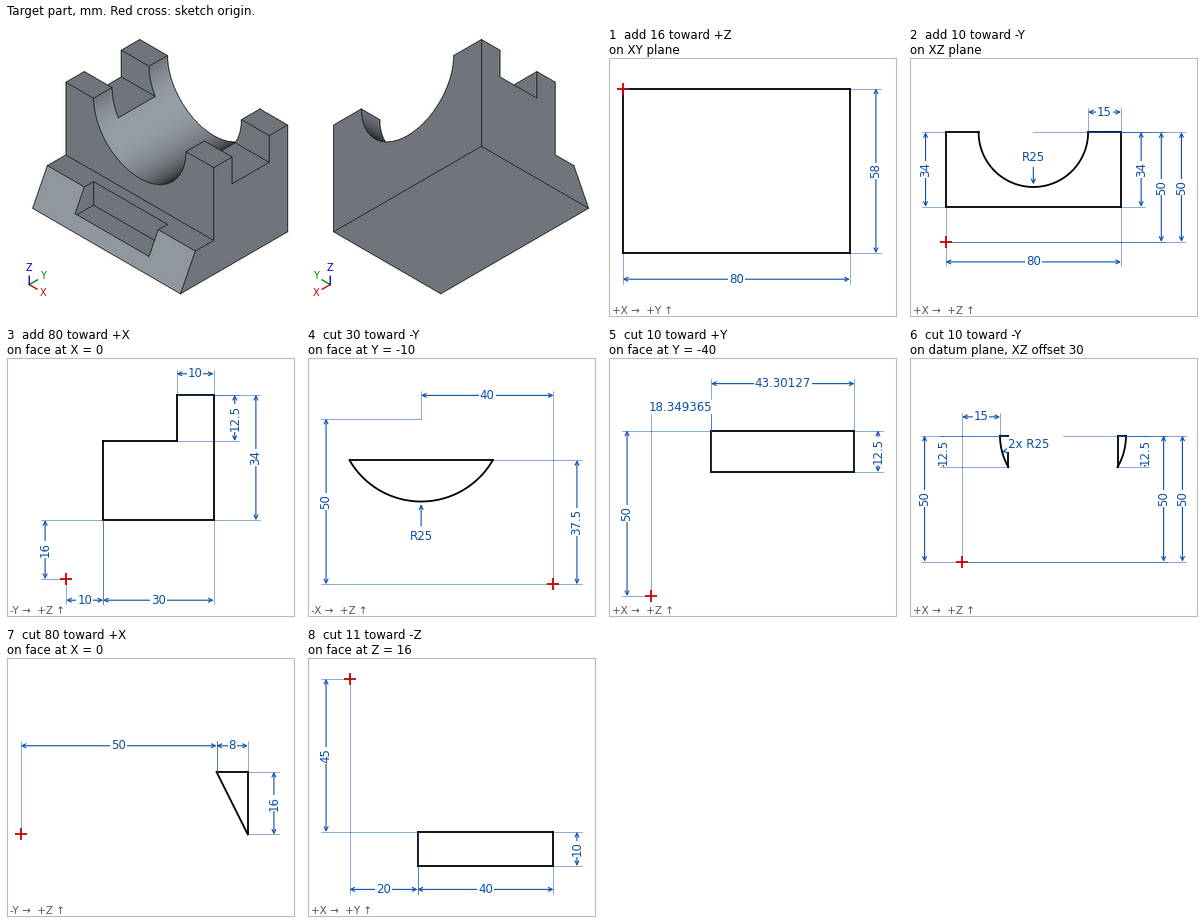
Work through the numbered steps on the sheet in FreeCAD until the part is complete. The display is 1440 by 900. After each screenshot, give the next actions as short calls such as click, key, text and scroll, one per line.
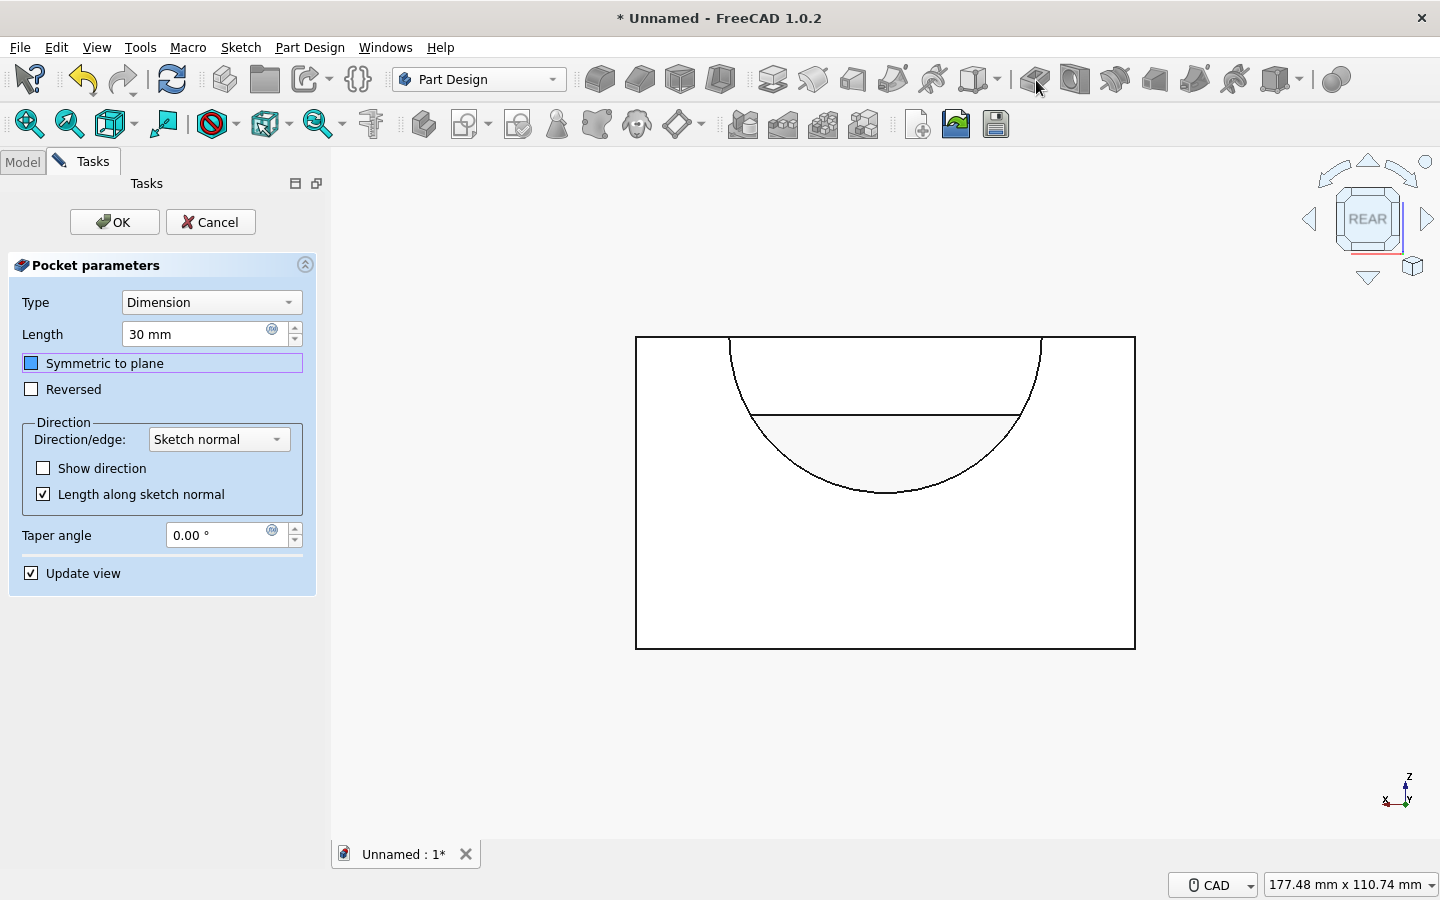
click(115, 222)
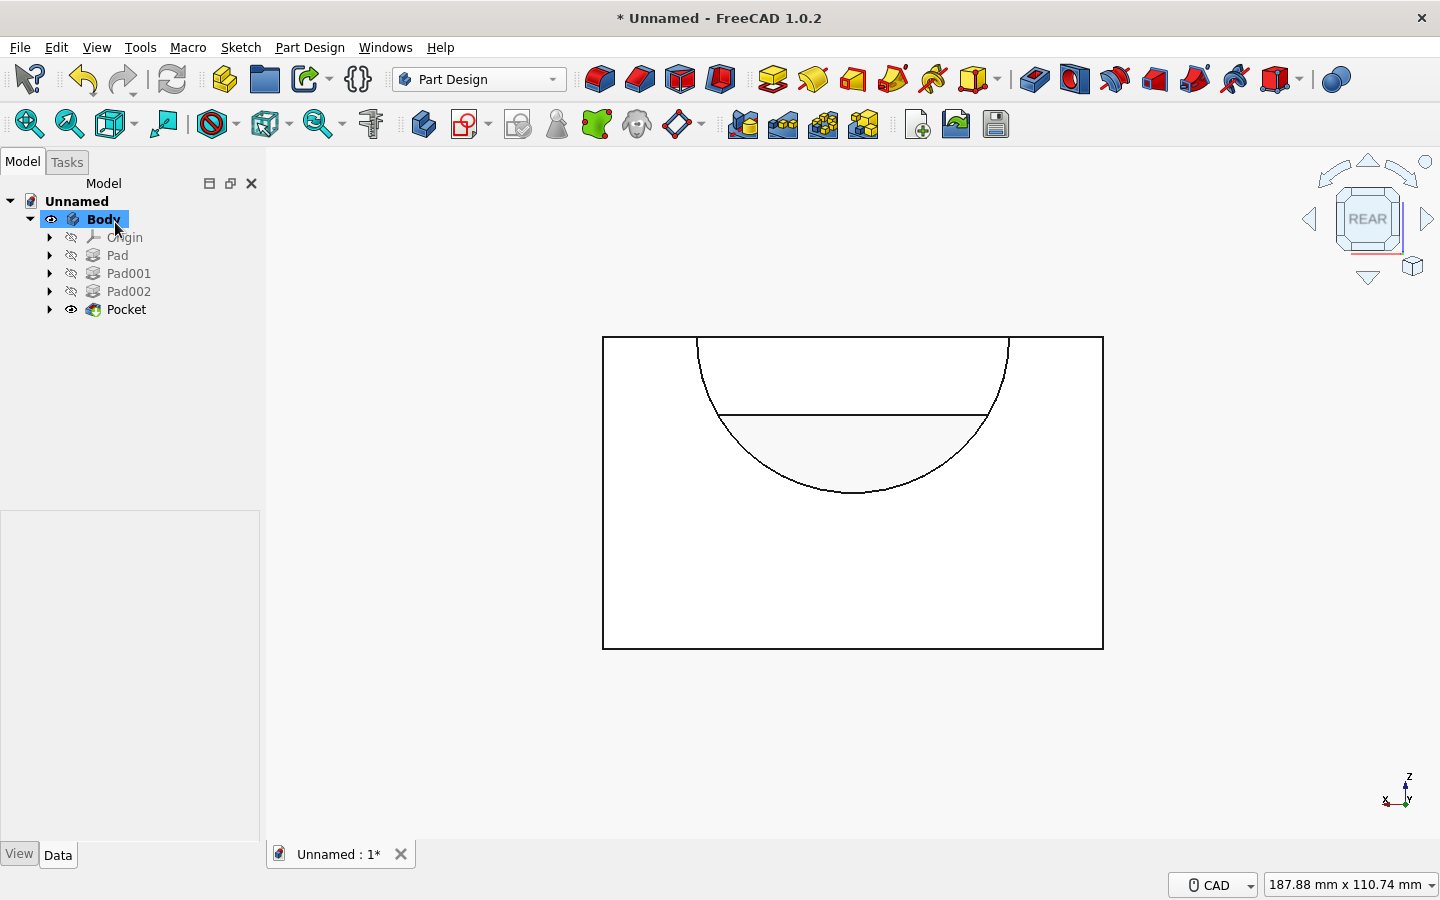
key(0)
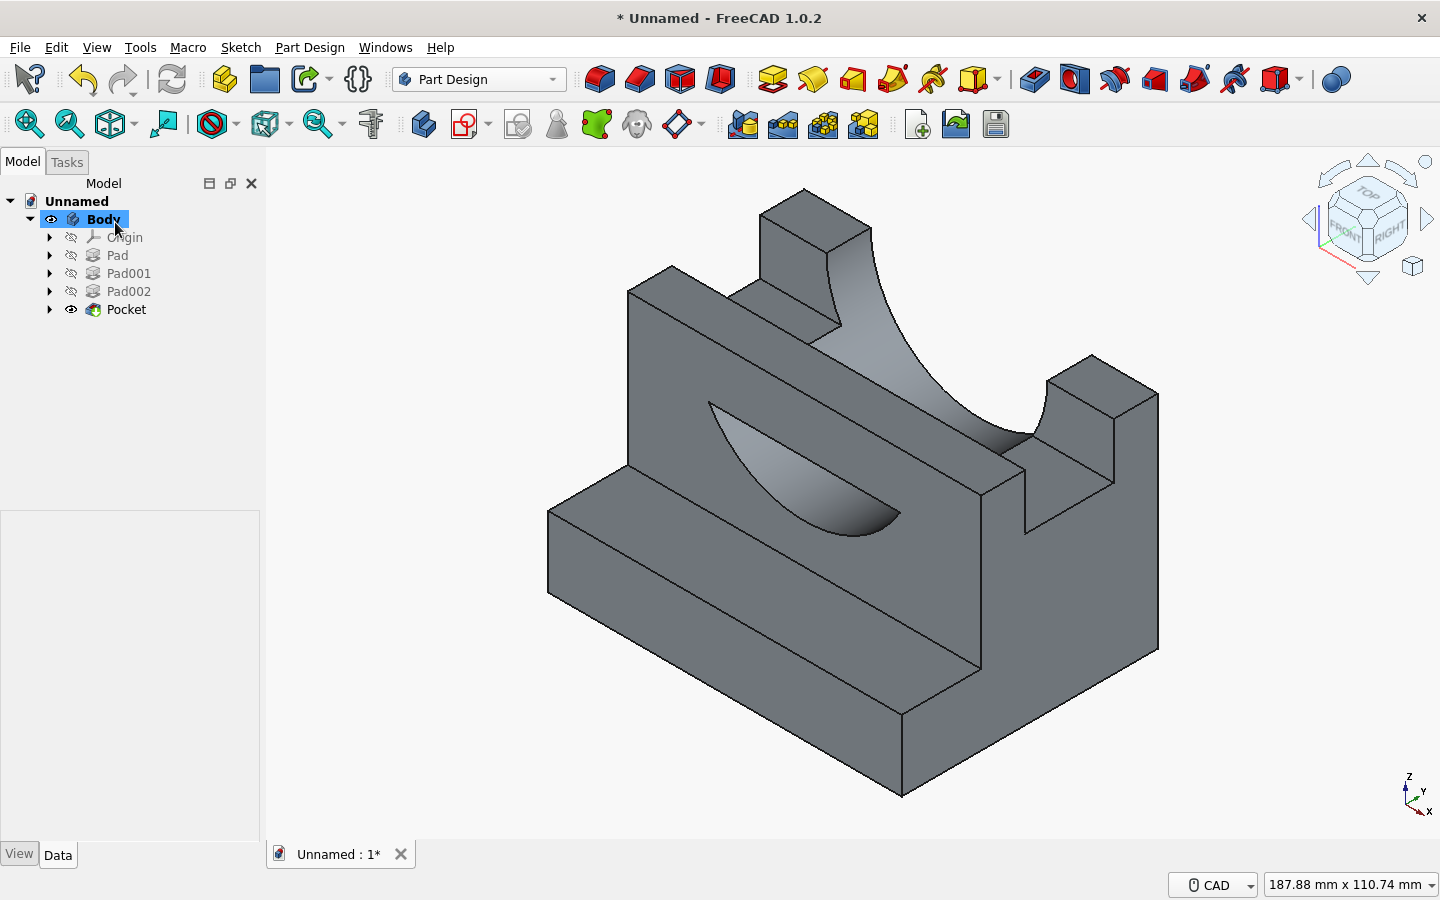
click(905, 587)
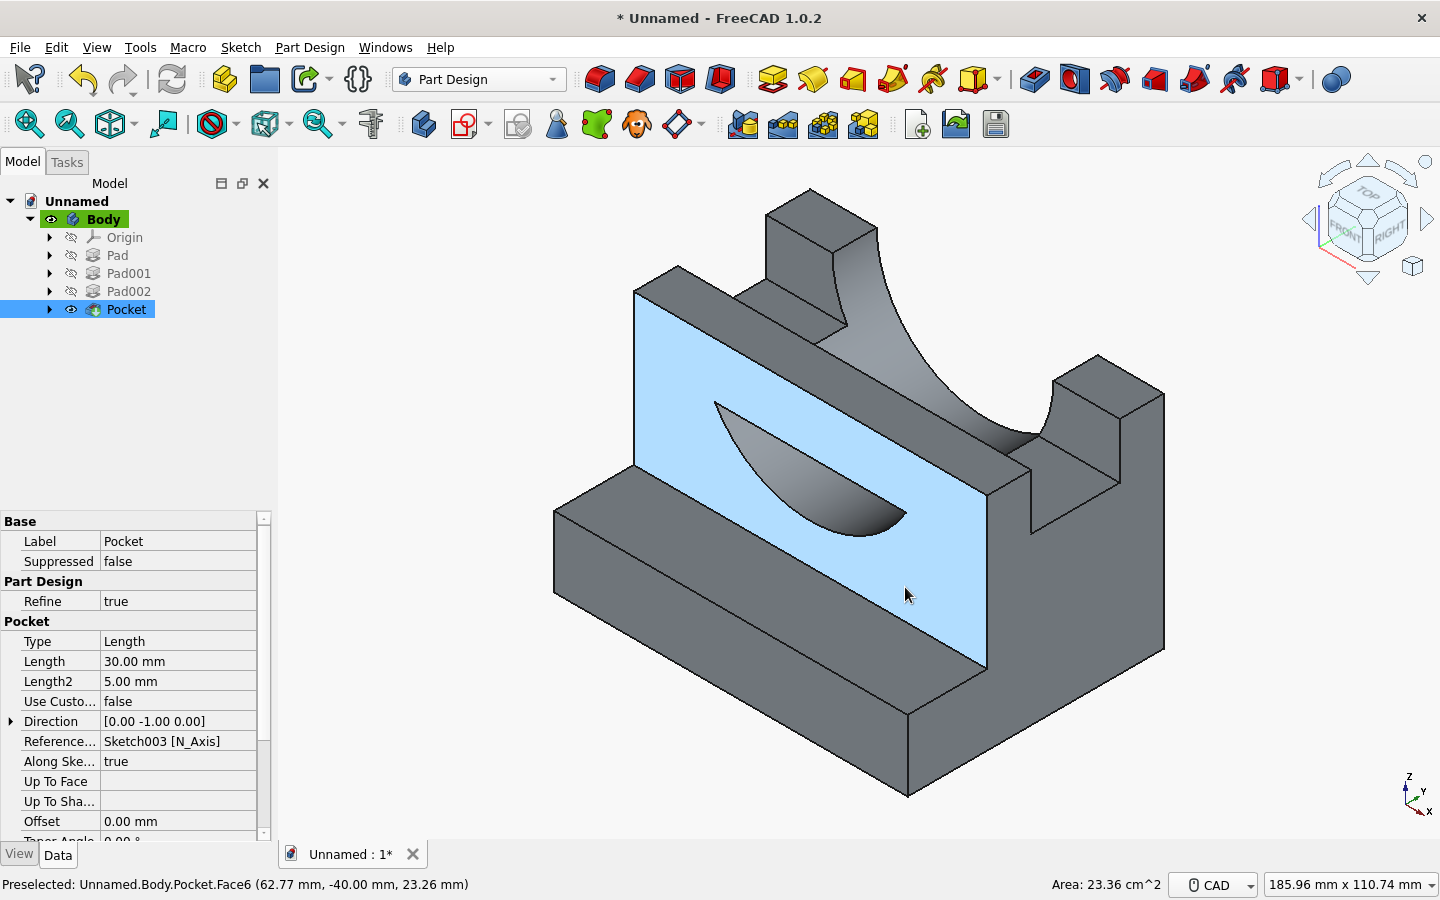
click(464, 124)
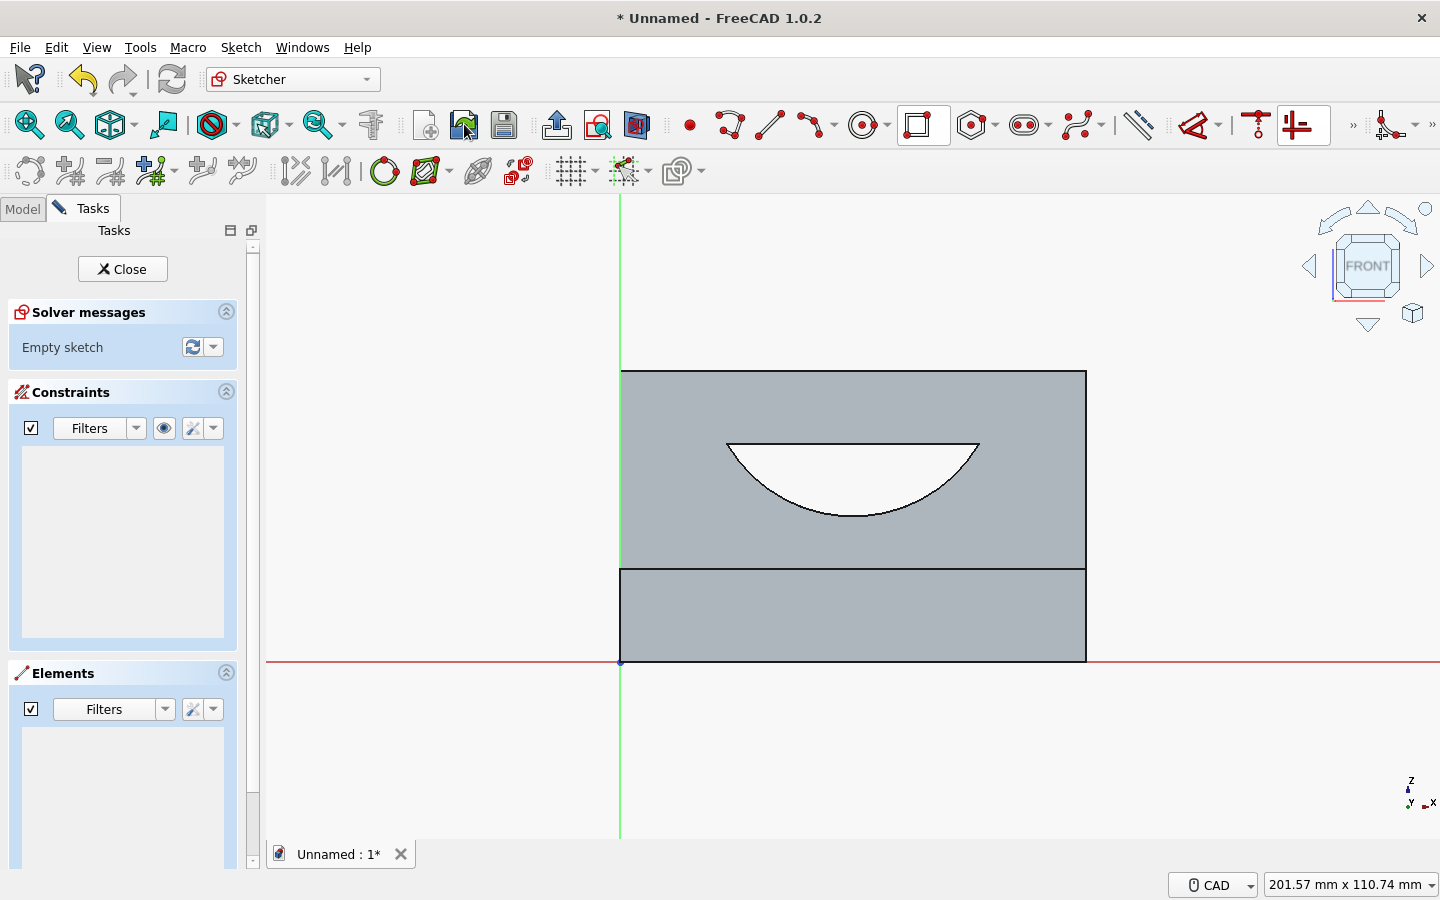
scroll(830, 517, up, 2)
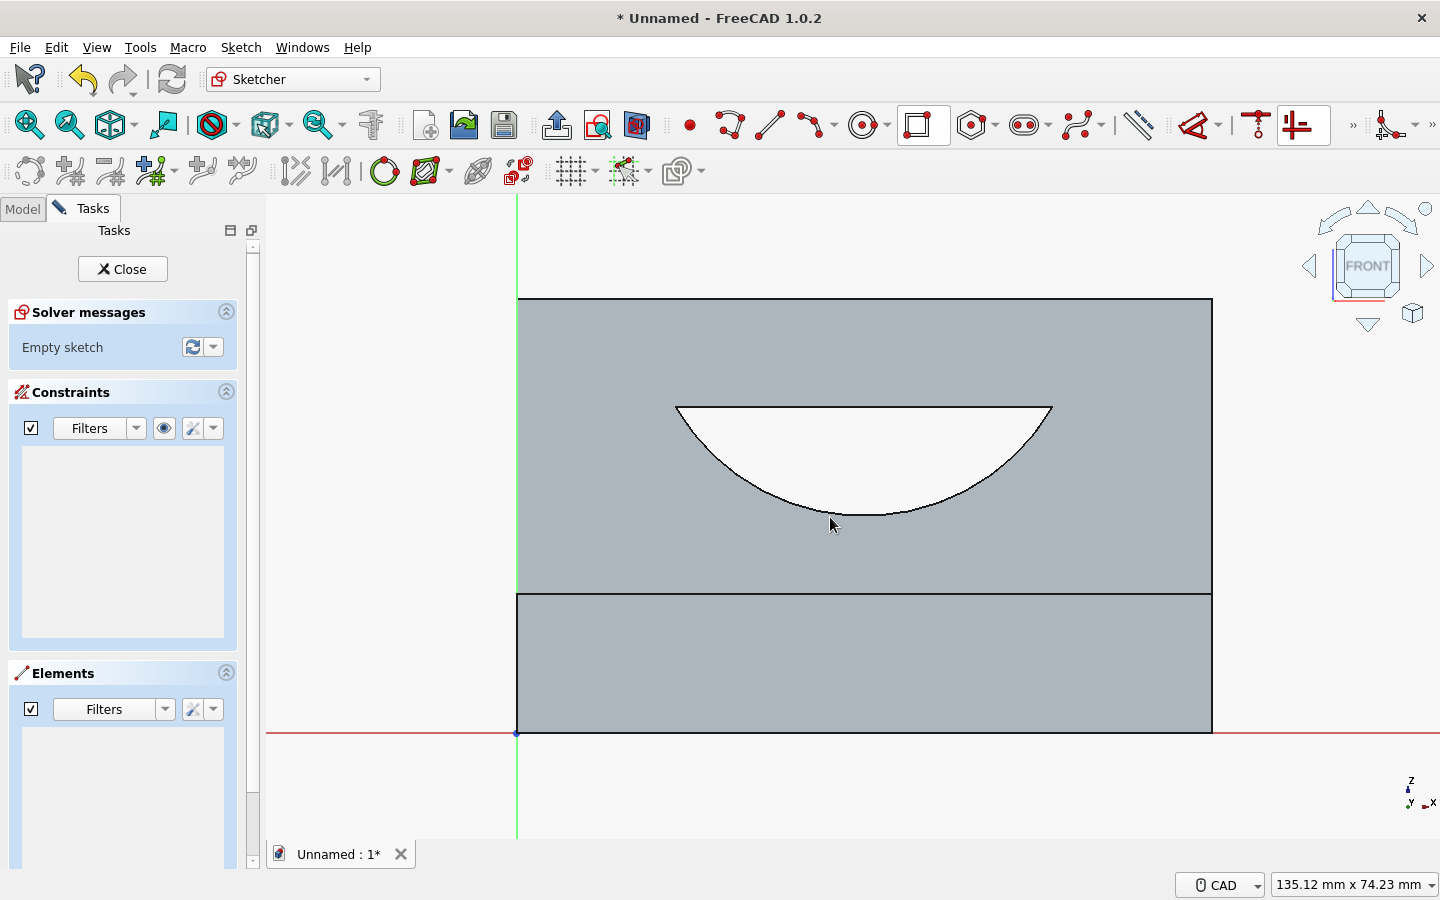
click(918, 126)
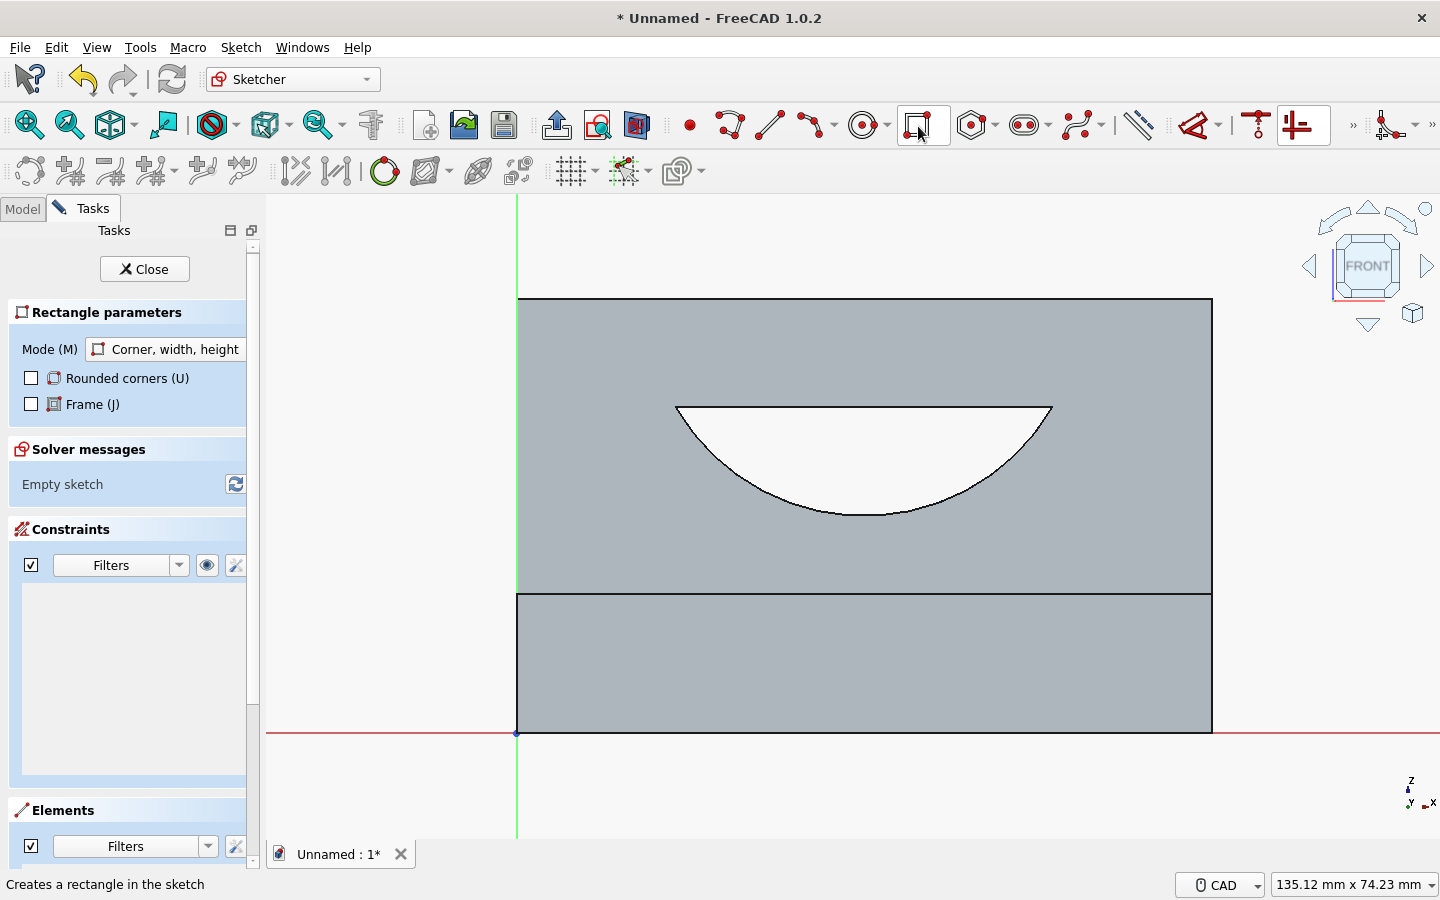
click(676, 299)
move(1052, 407)